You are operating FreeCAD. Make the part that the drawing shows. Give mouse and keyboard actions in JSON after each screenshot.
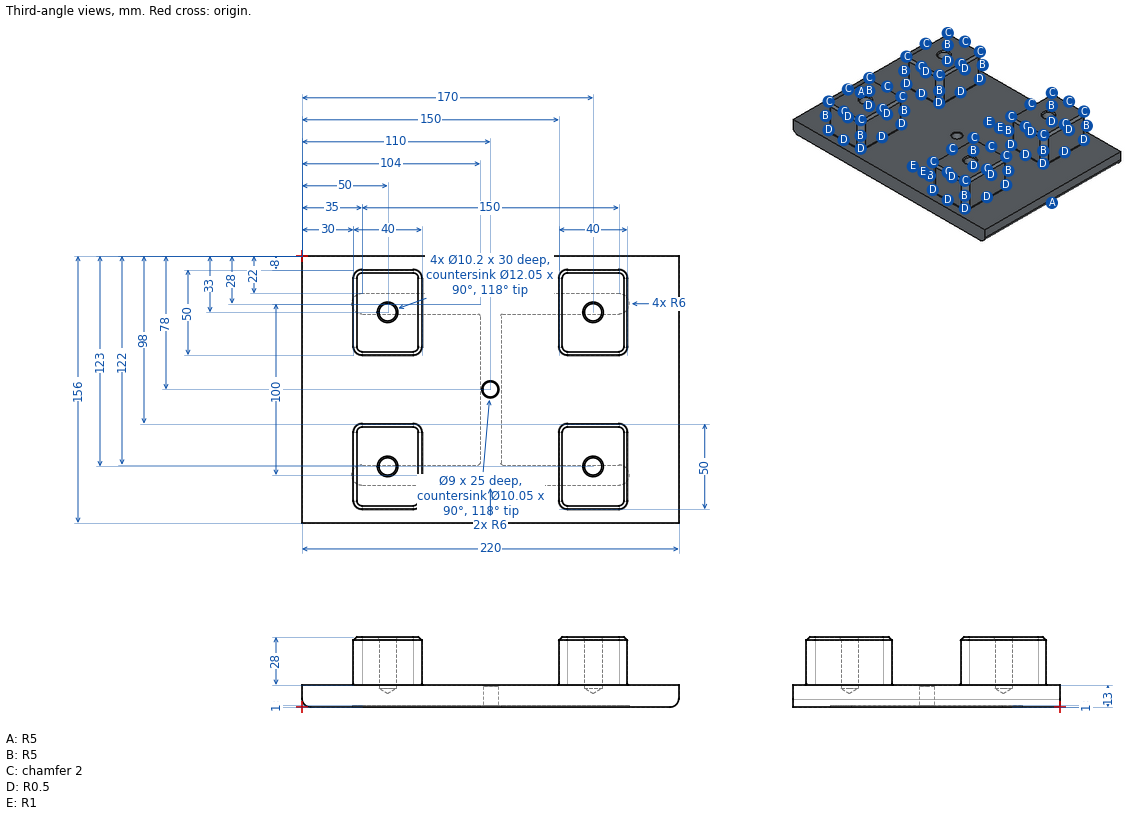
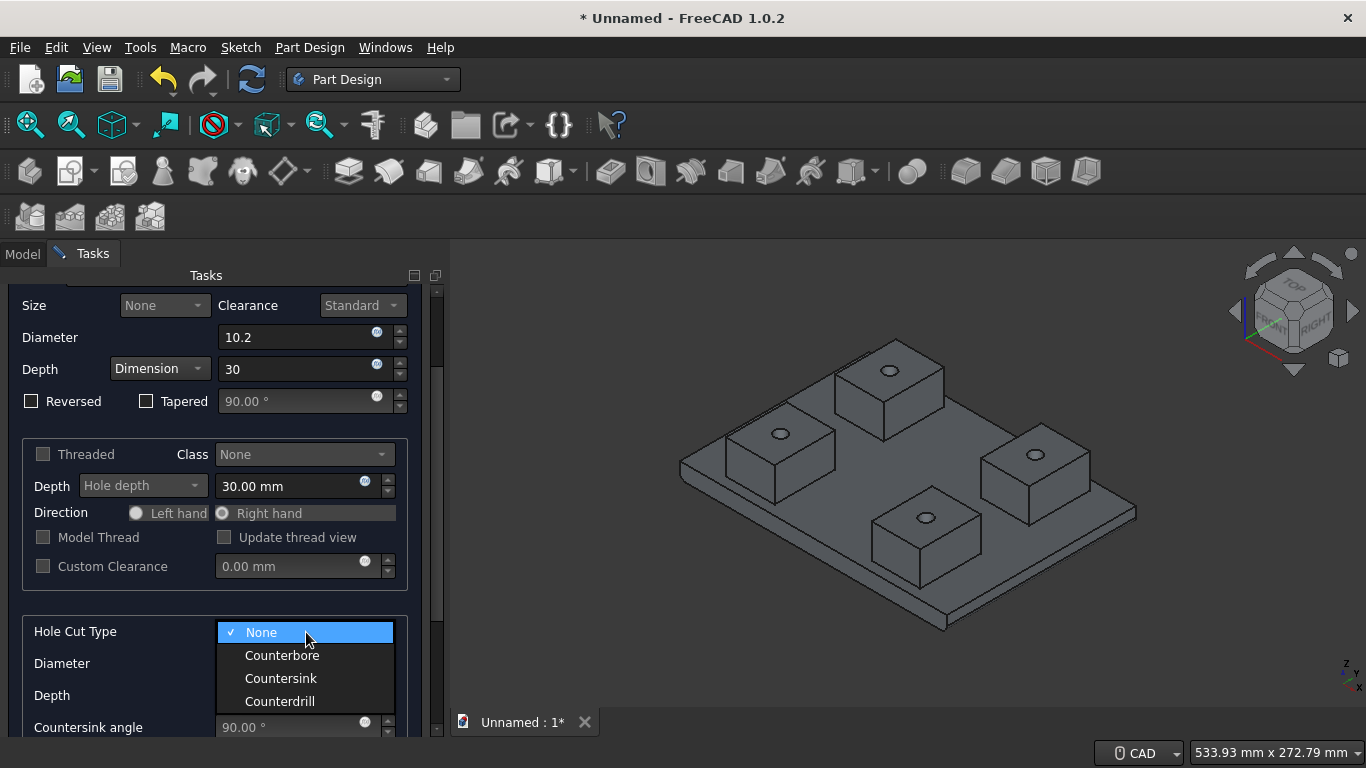
{"action": "left_click", "coordinate": [304, 678]}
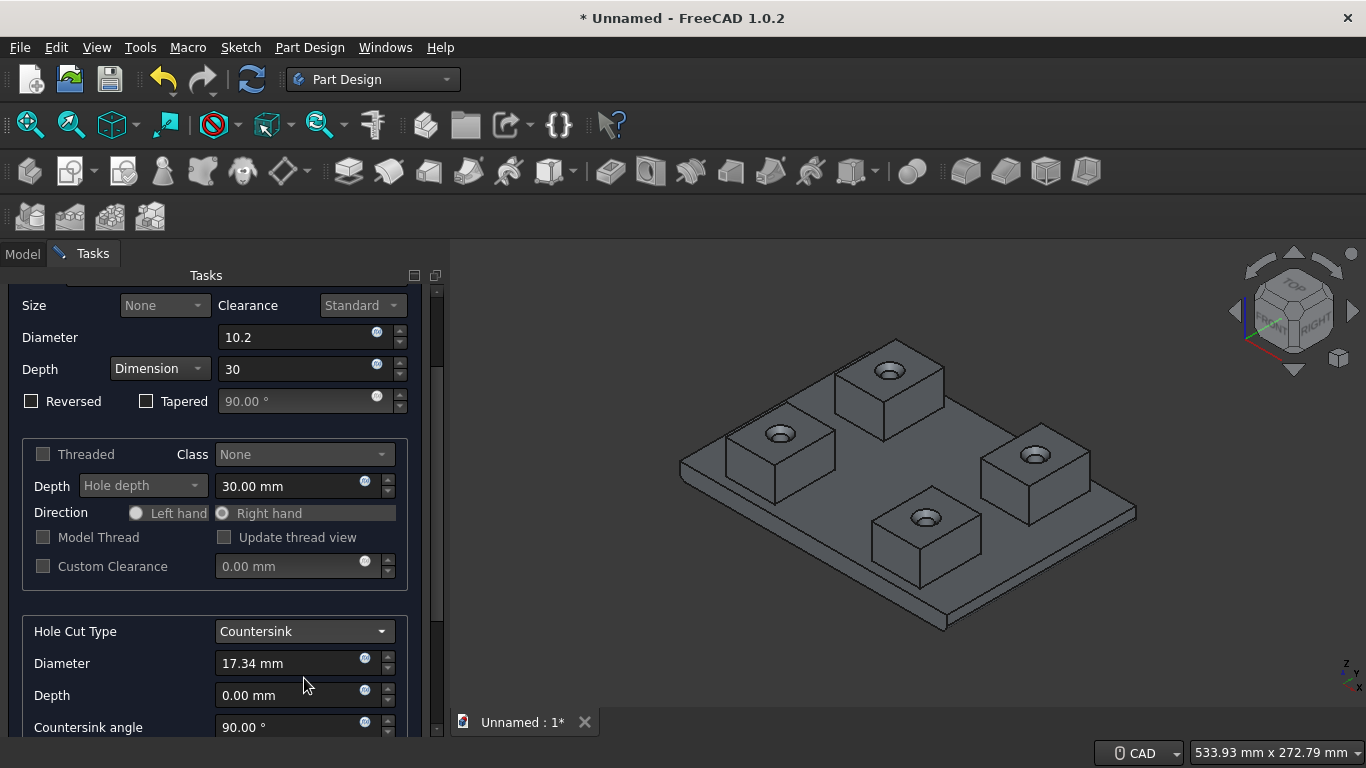
{"action": "triple_click", "coordinate": [298, 663]}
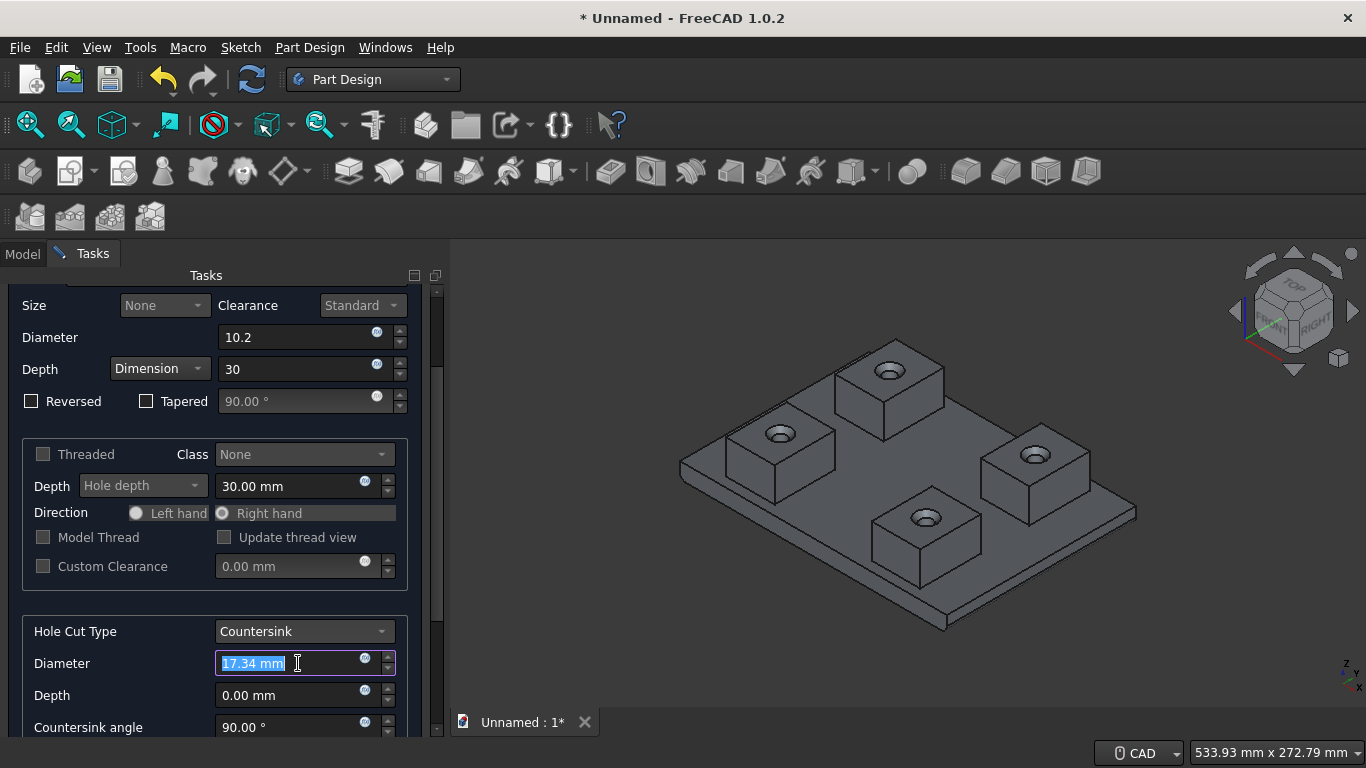
{"action": "type", "text": "12.05"}
{"action": "key", "text": "Tab"}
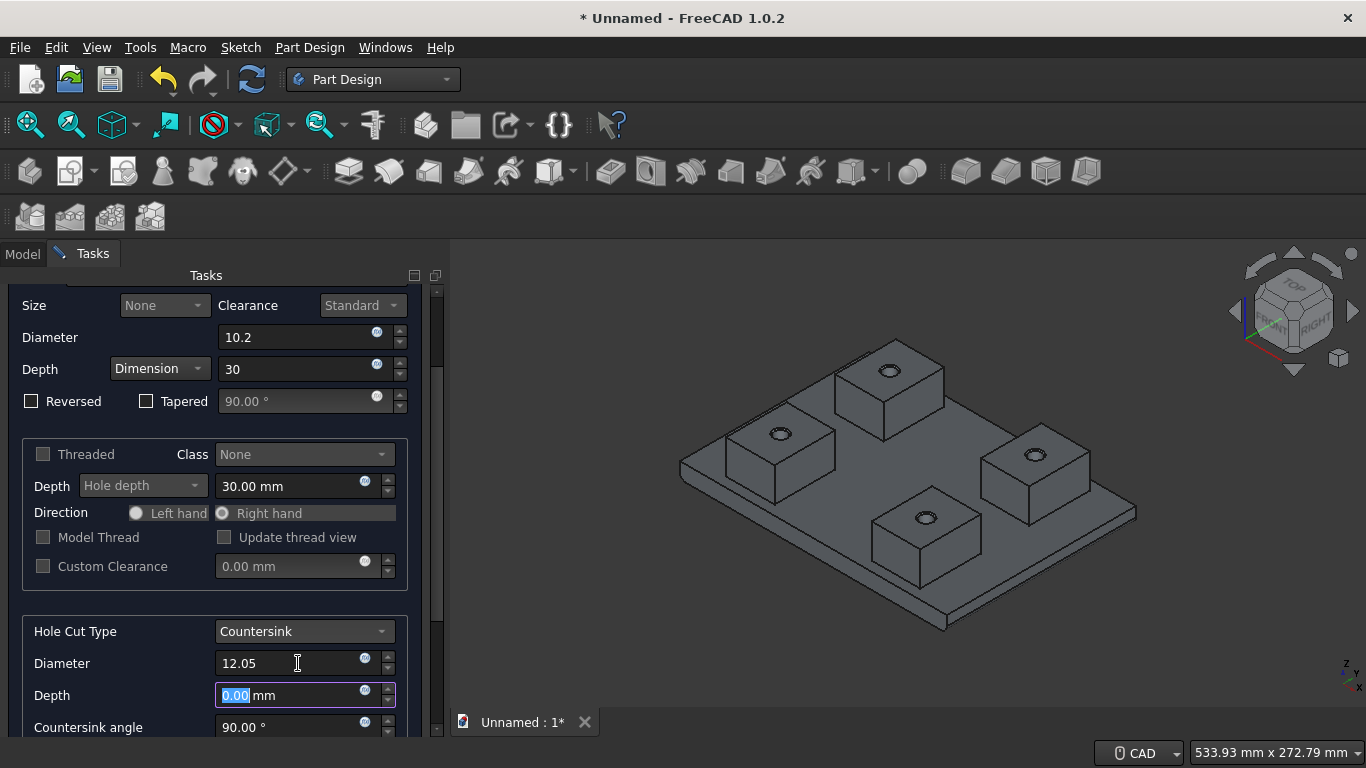
{"action": "scroll", "coordinate": [437, 510], "scroll_direction": "up", "scroll_amount": 3}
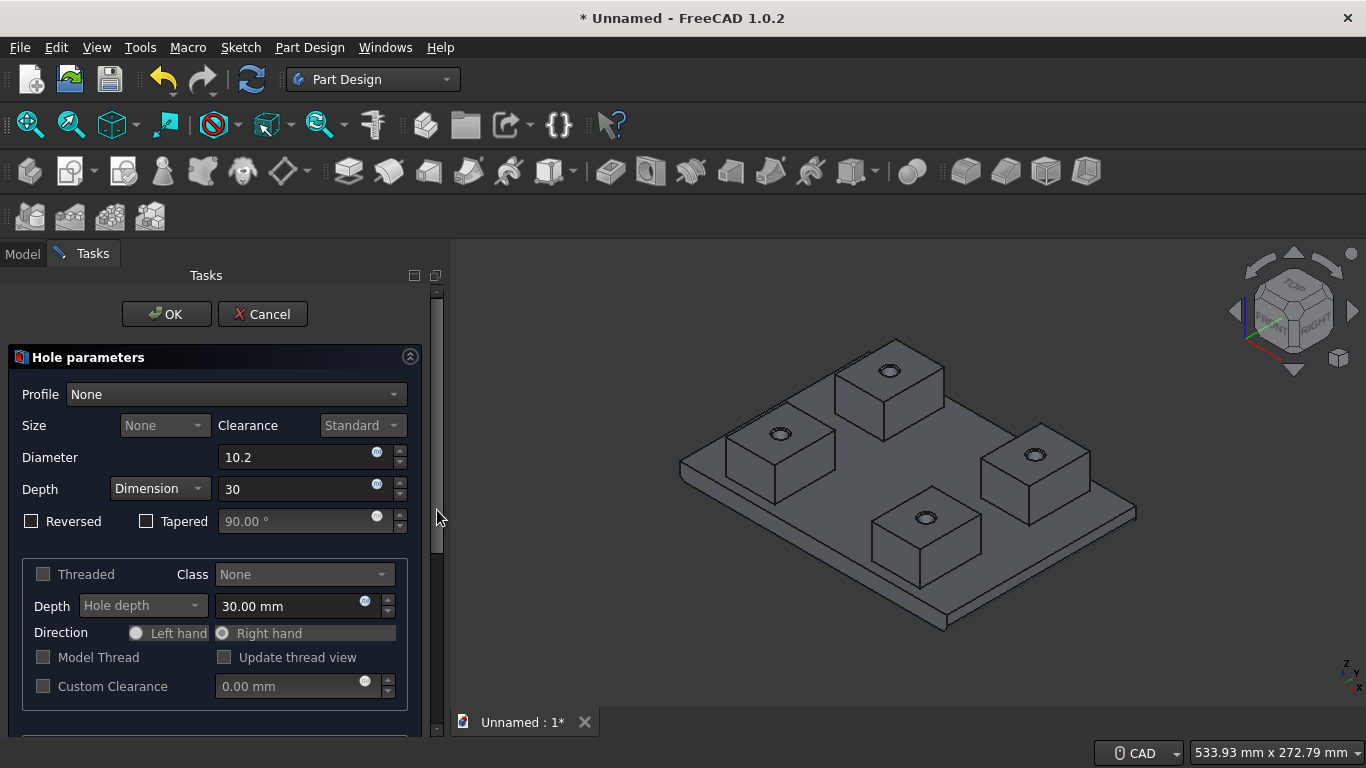
{"action": "left_click", "coordinate": [167, 314]}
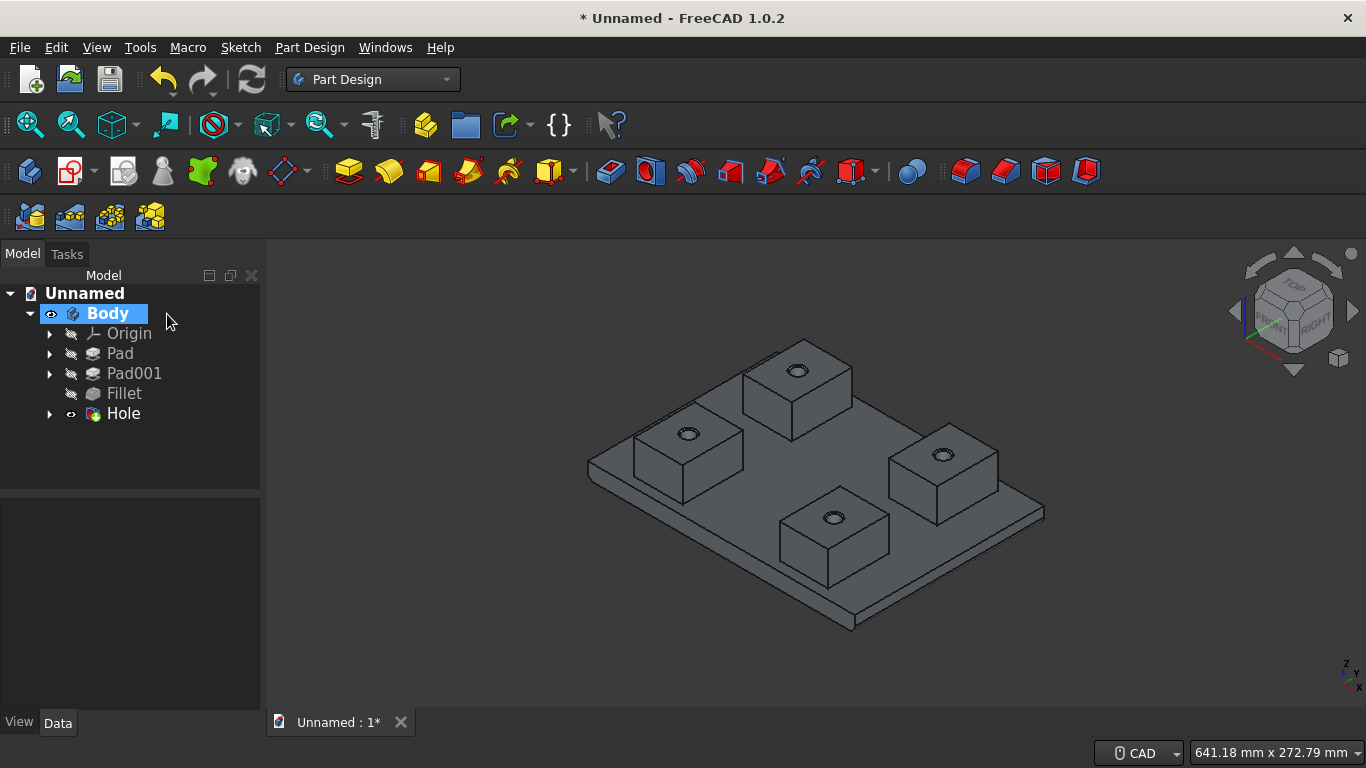
{"action": "left_click", "coordinate": [816, 483]}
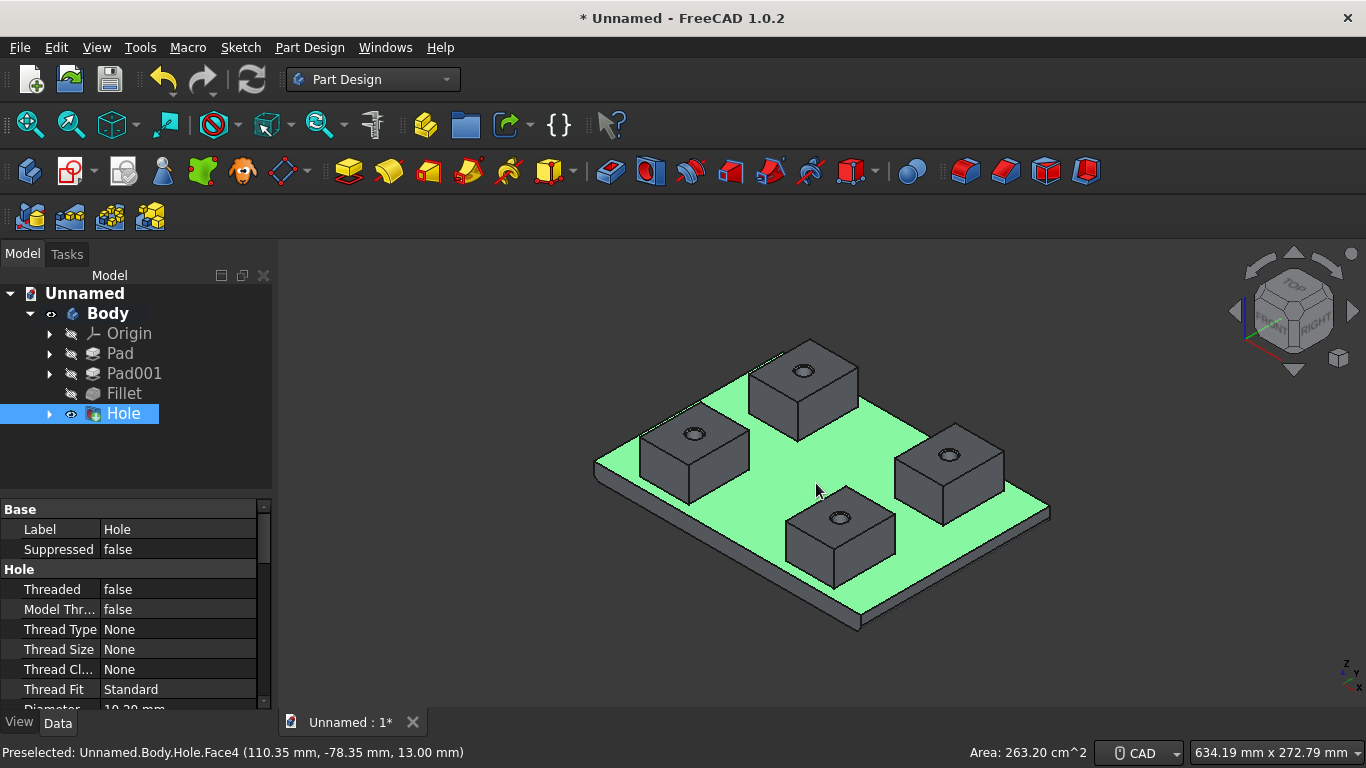
{"action": "left_click", "coordinate": [70, 172]}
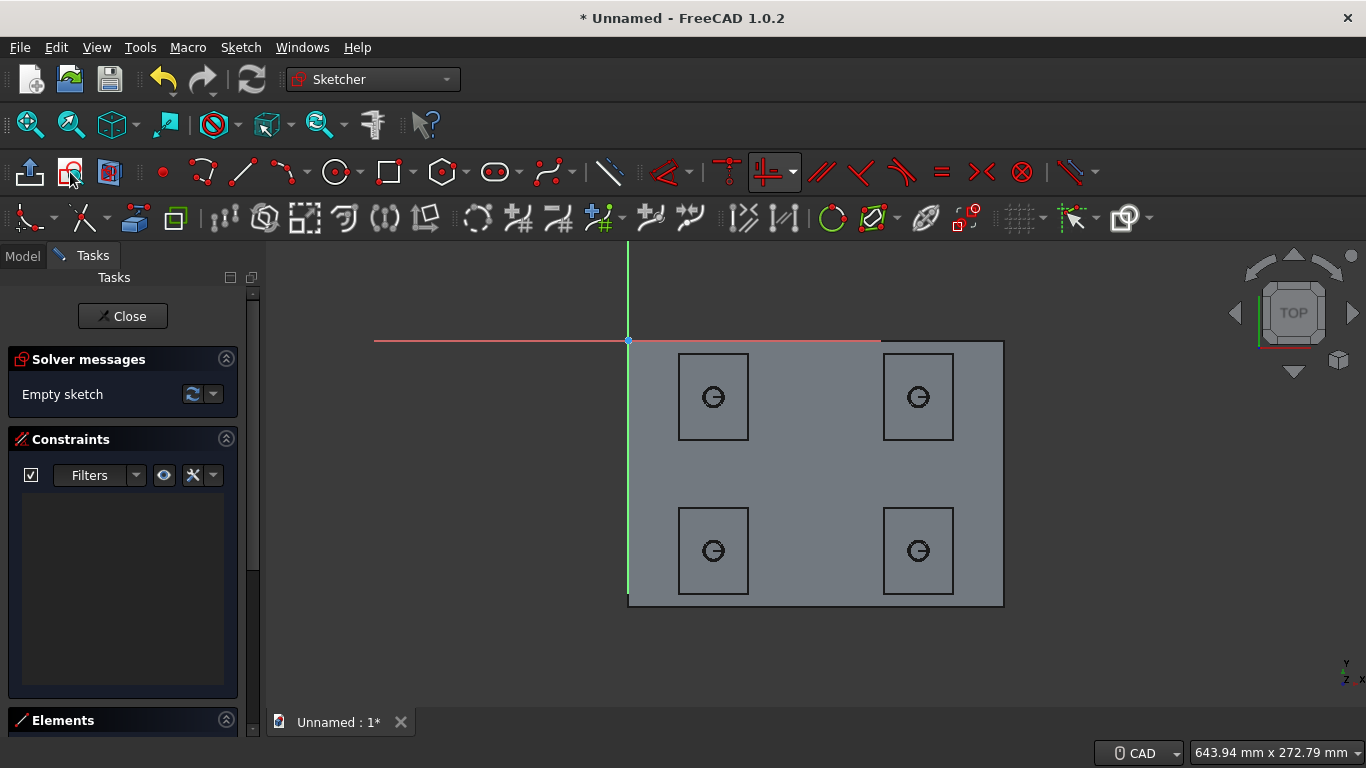
{"action": "scroll", "coordinate": [820, 474], "scroll_direction": "up", "scroll_amount": 15}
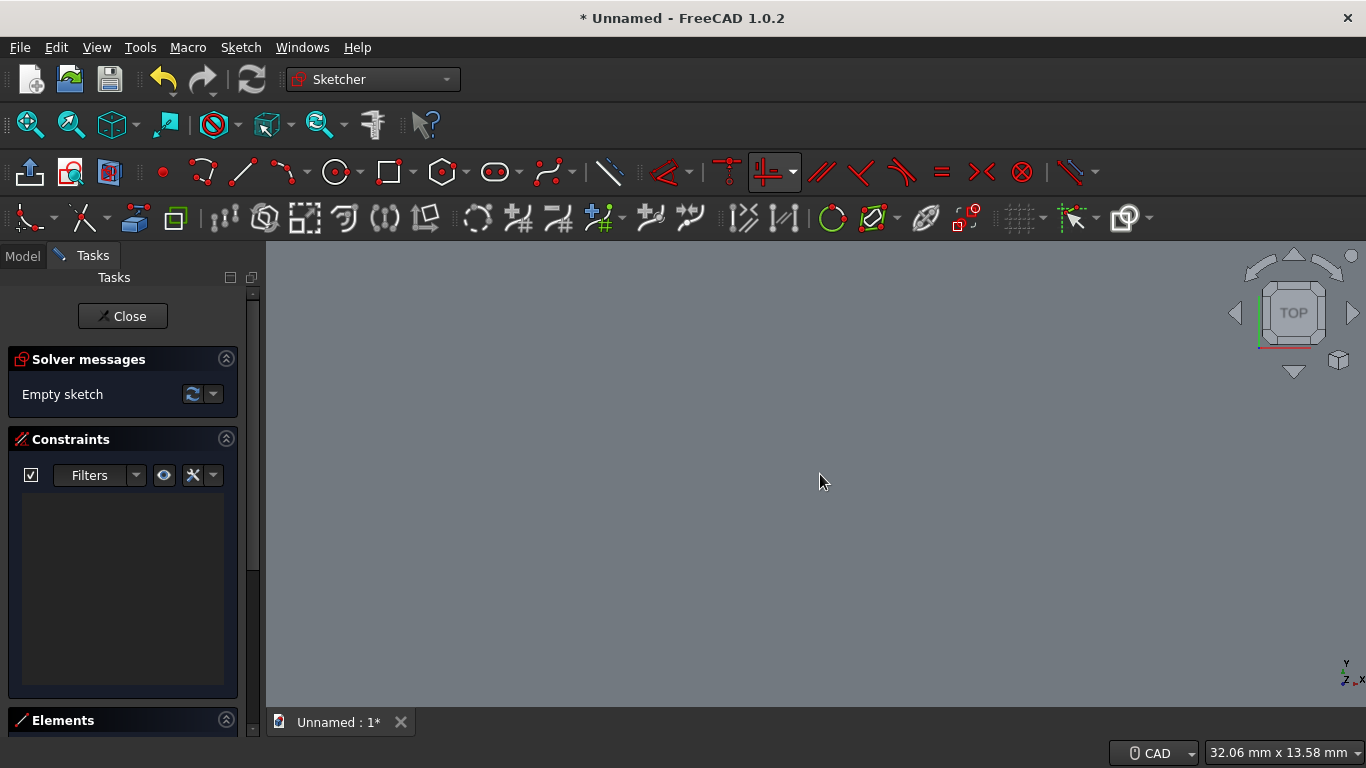
{"action": "key", "text": "g c"}